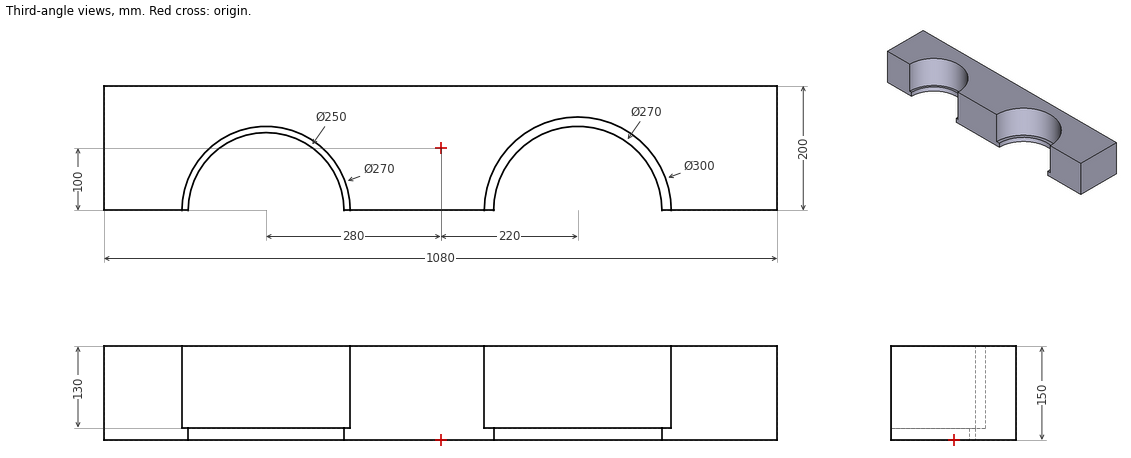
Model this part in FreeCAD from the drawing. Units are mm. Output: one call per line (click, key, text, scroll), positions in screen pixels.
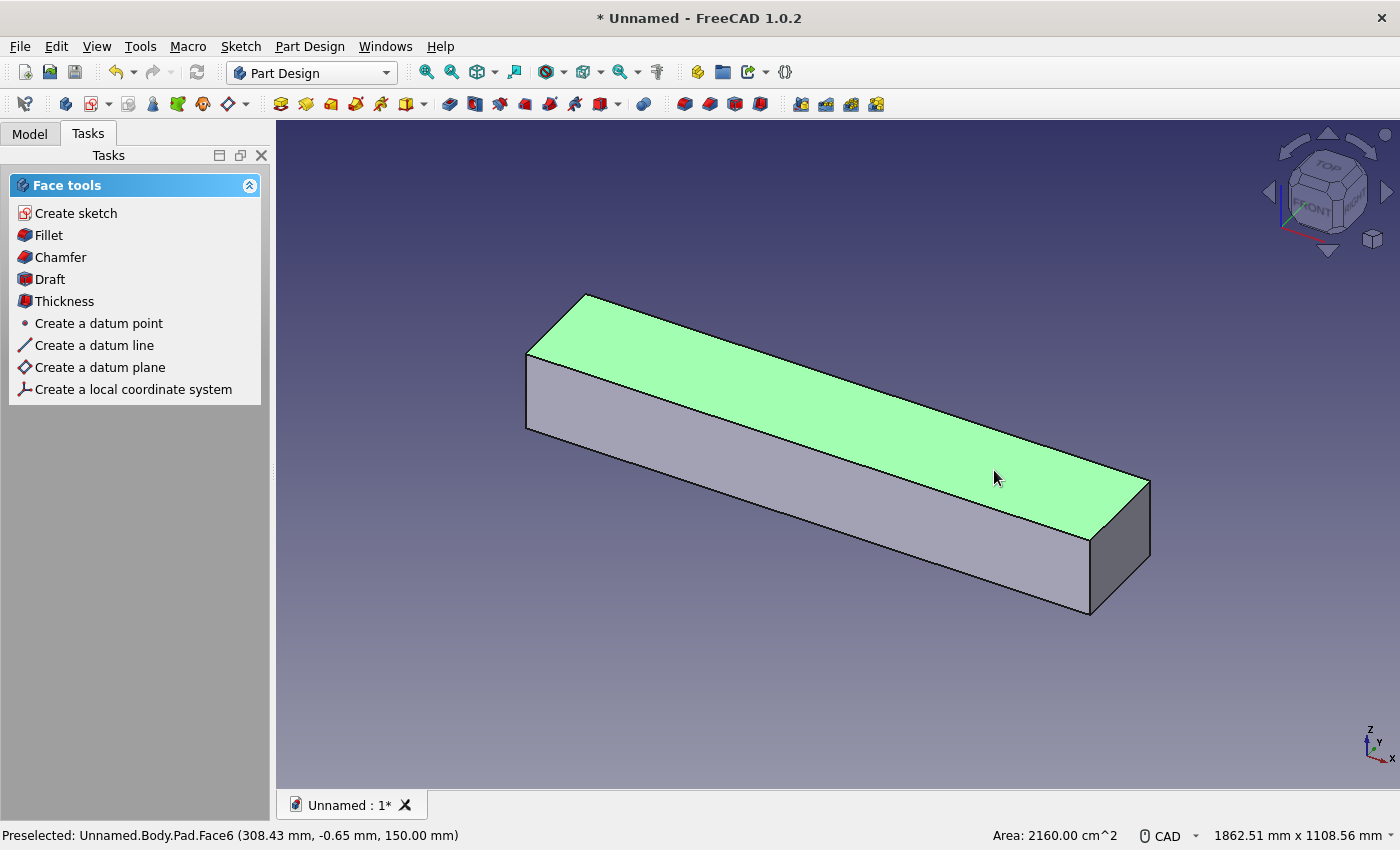
click(90, 104)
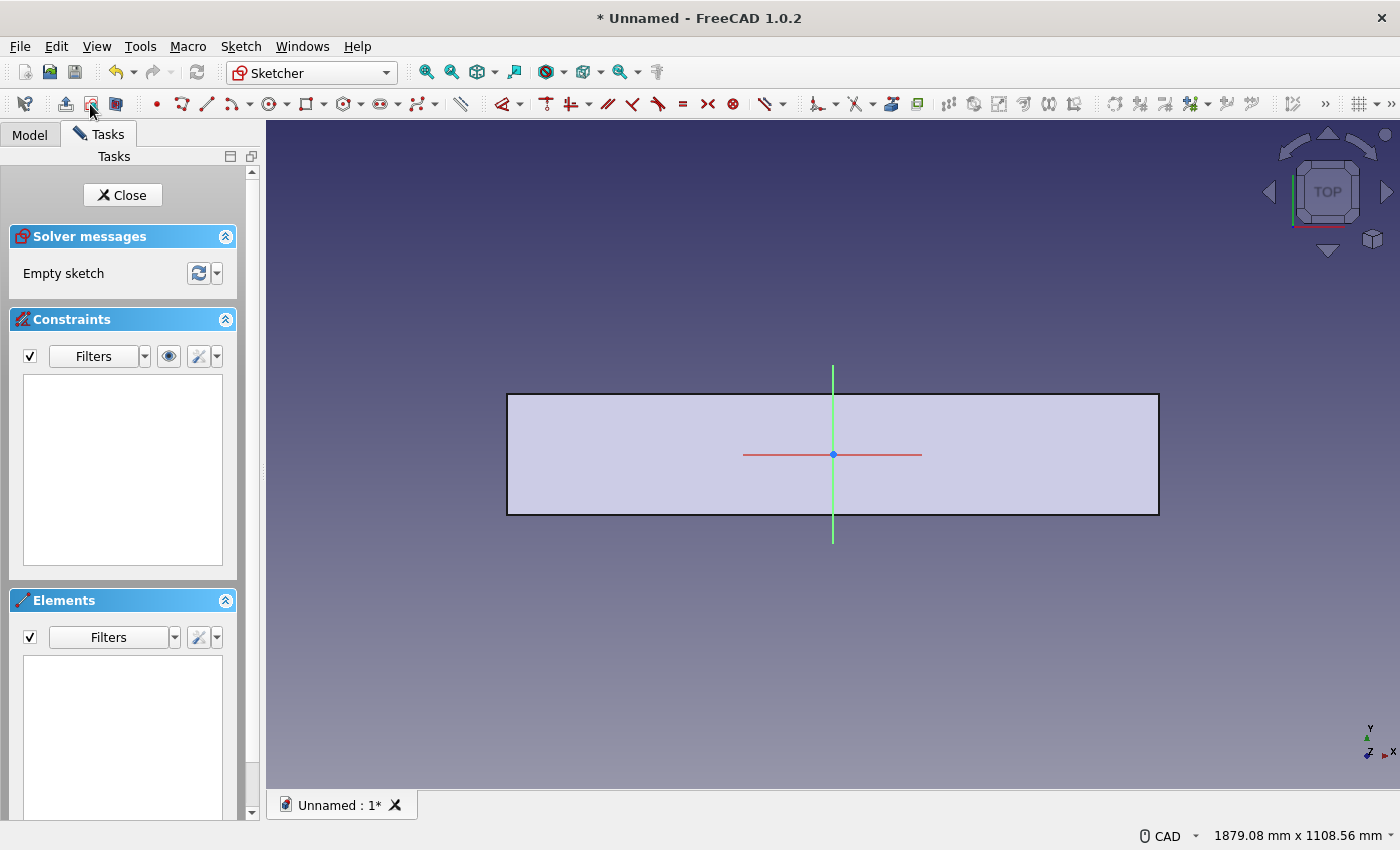
scroll(931, 638, up, 2)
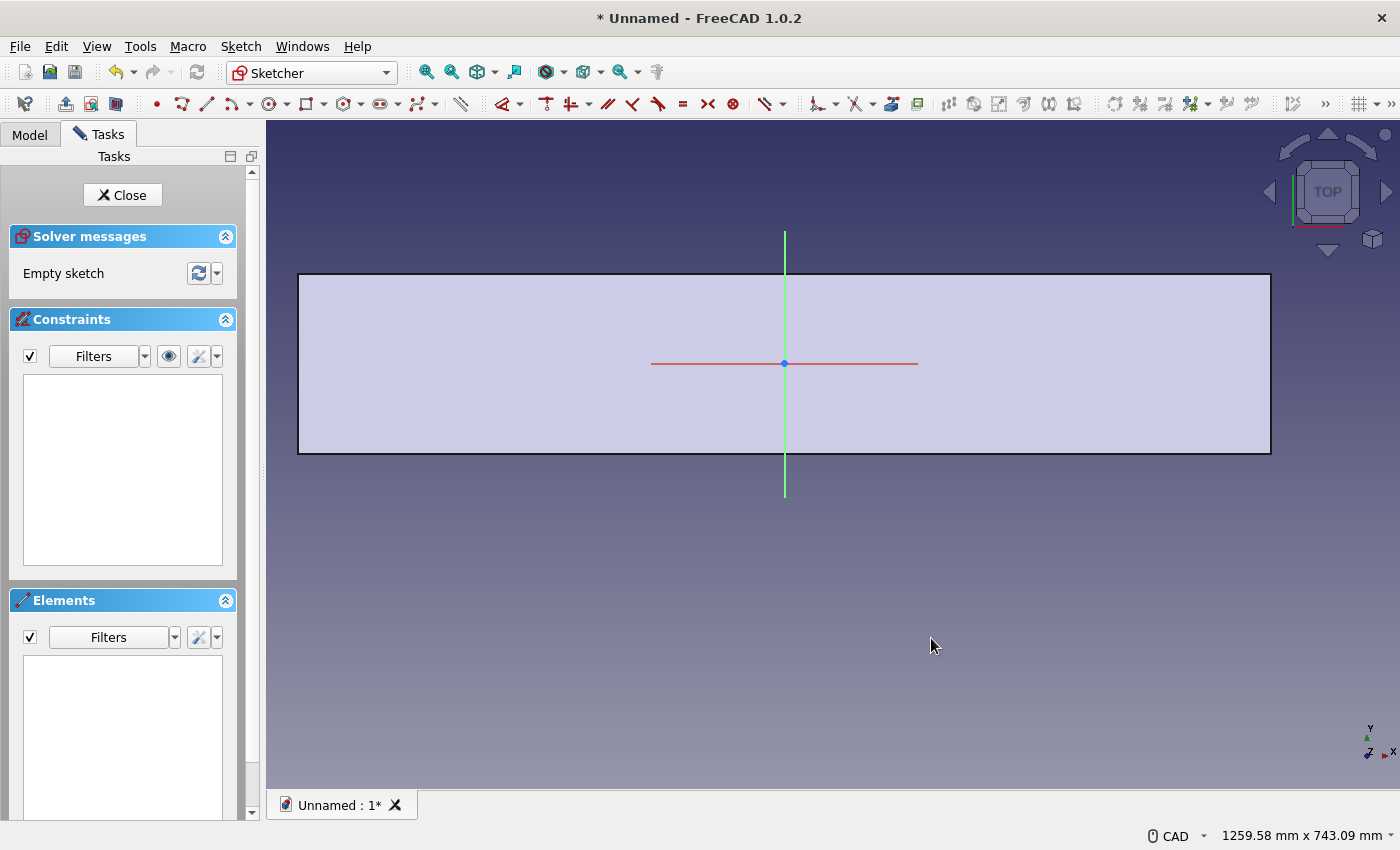
click(268, 104)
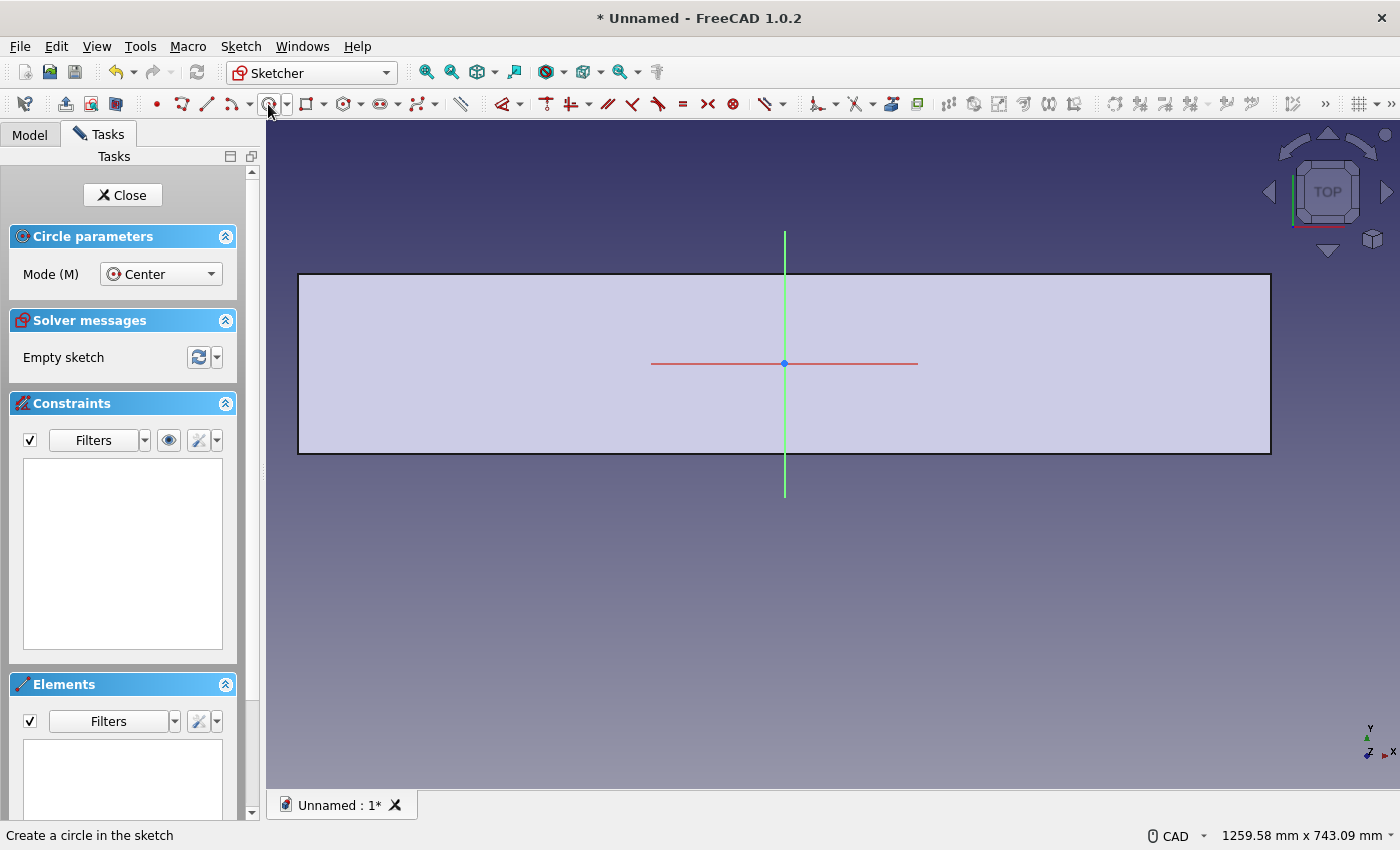
click(532, 454)
click(618, 540)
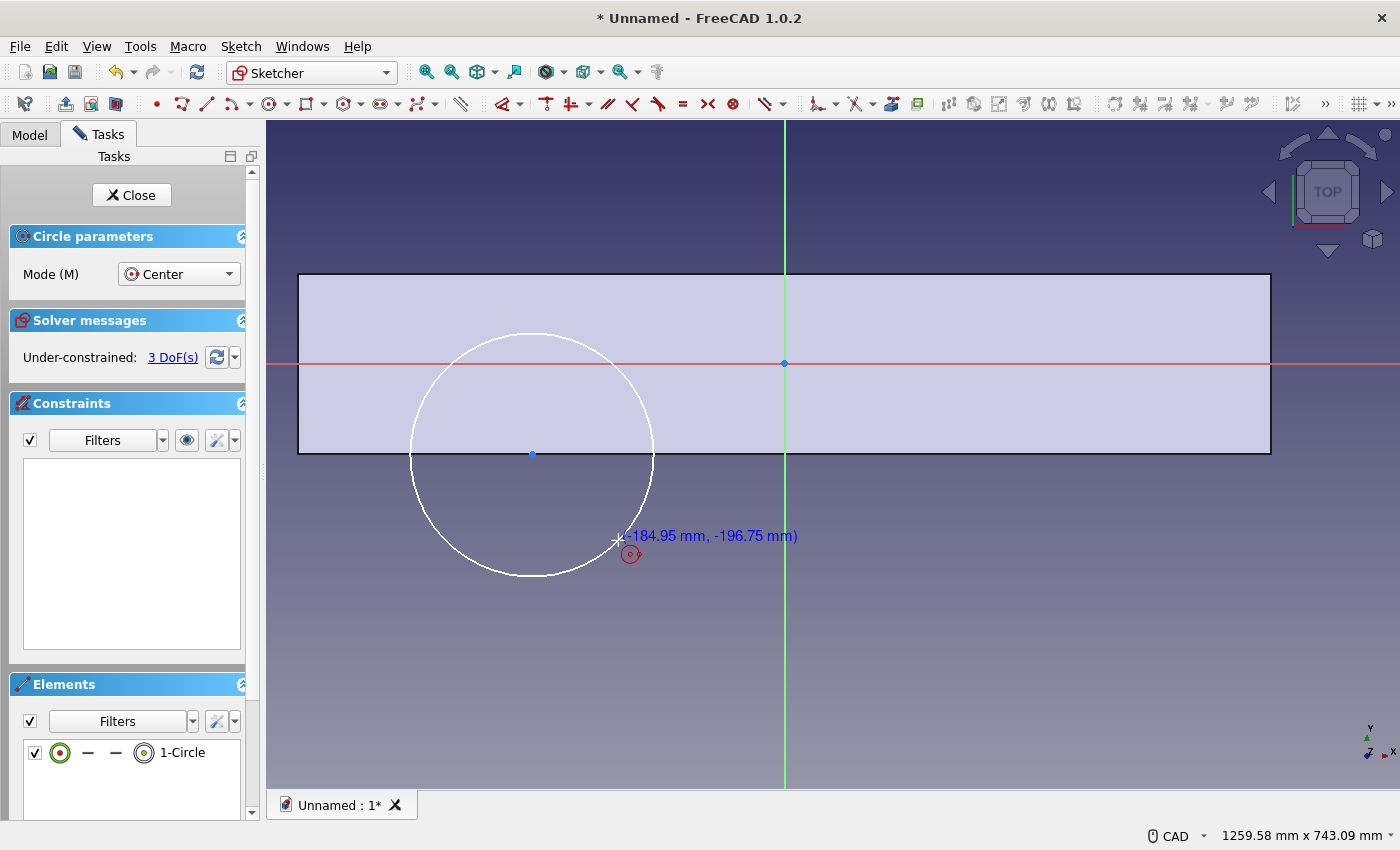
click(983, 454)
click(1078, 549)
key(Escape)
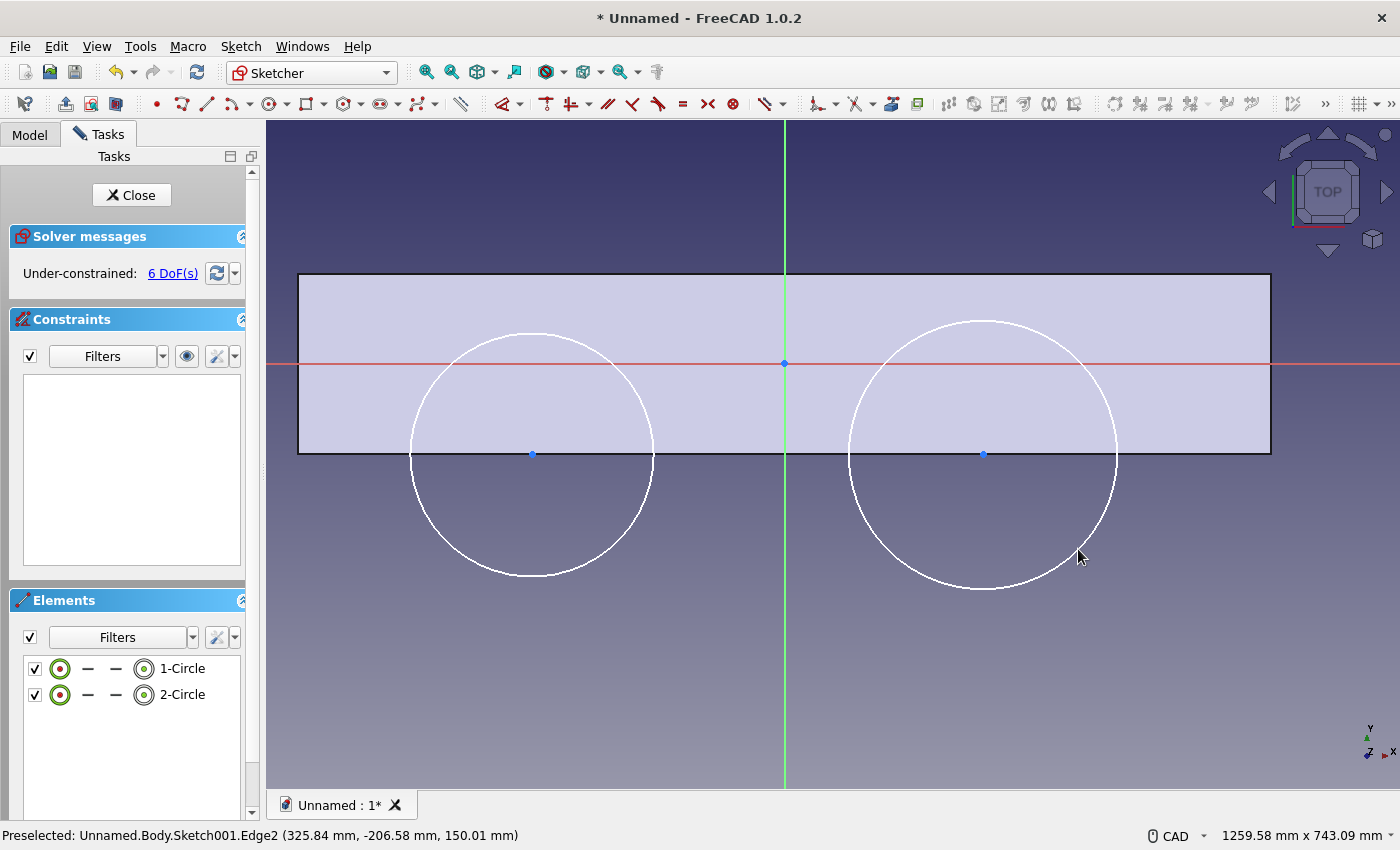
click(532, 455)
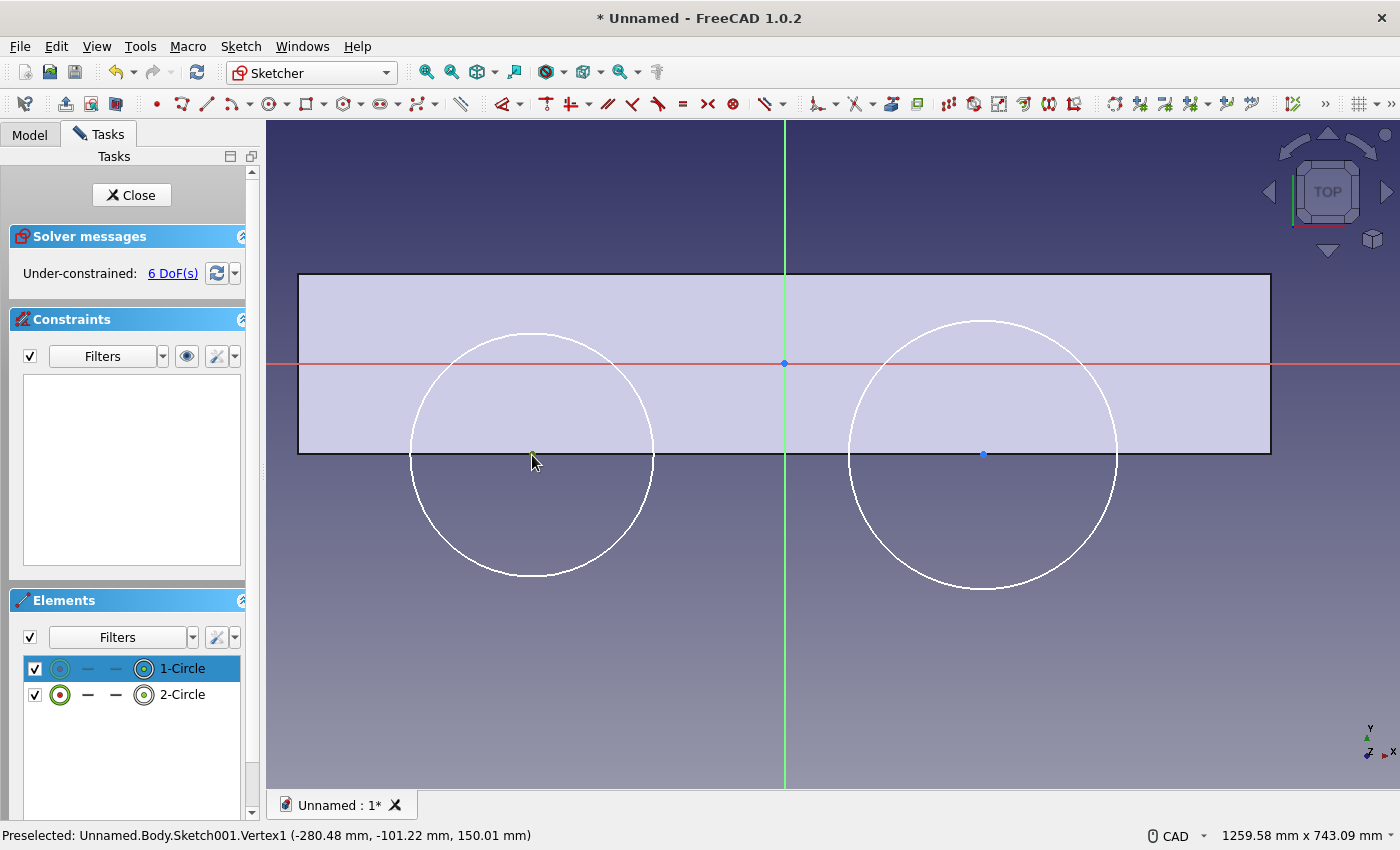
click(983, 455)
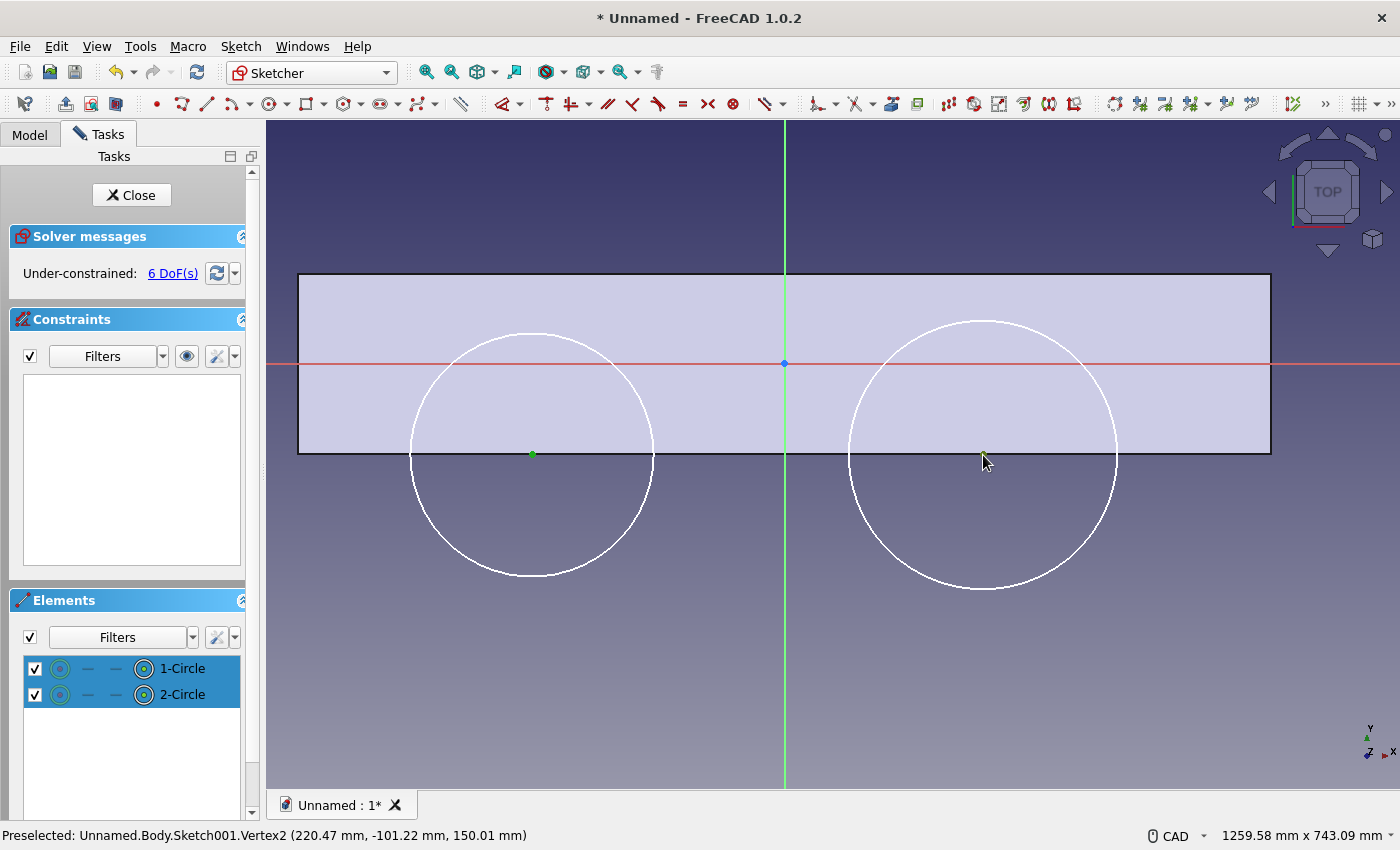
click(588, 104)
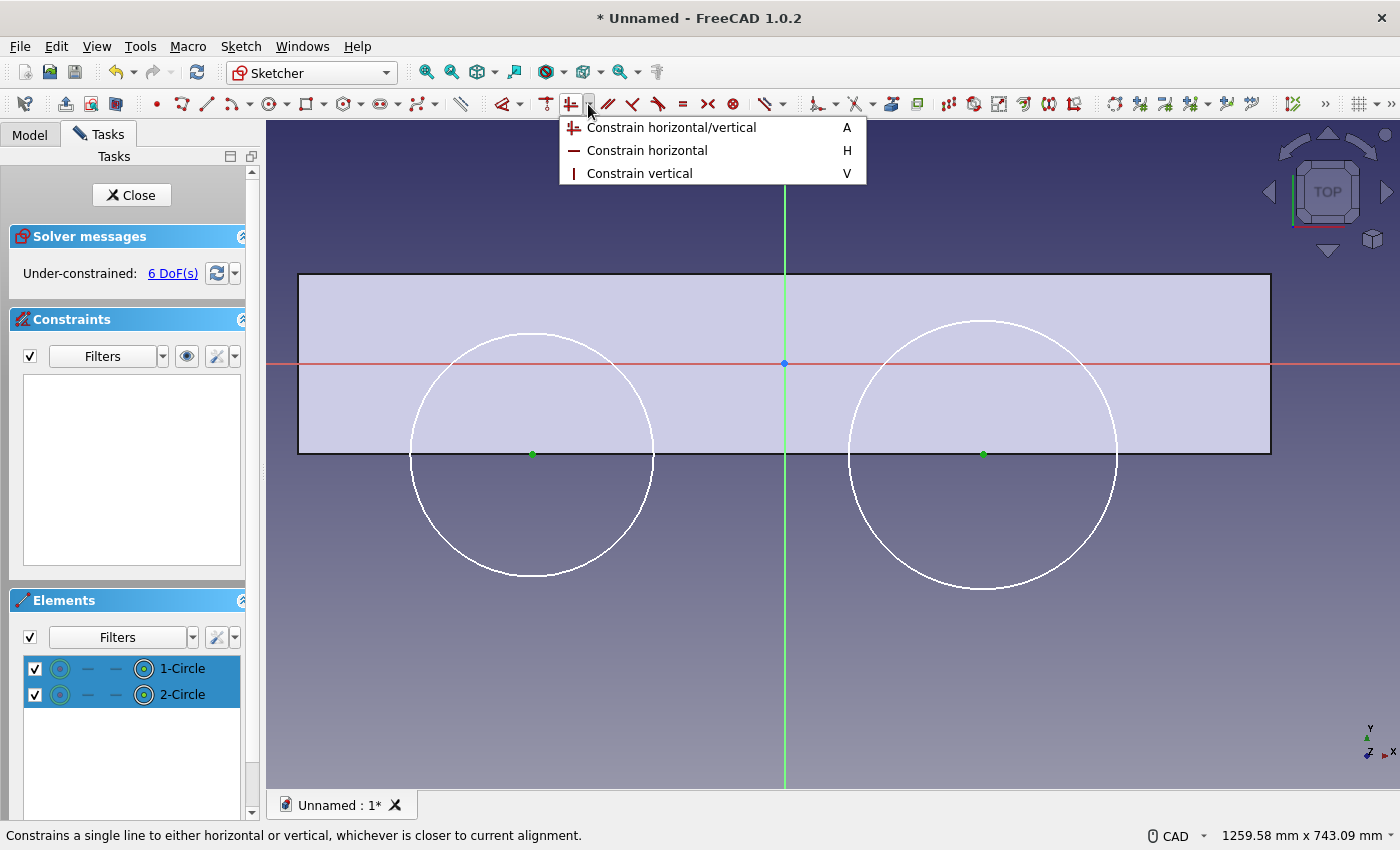
click(713, 150)